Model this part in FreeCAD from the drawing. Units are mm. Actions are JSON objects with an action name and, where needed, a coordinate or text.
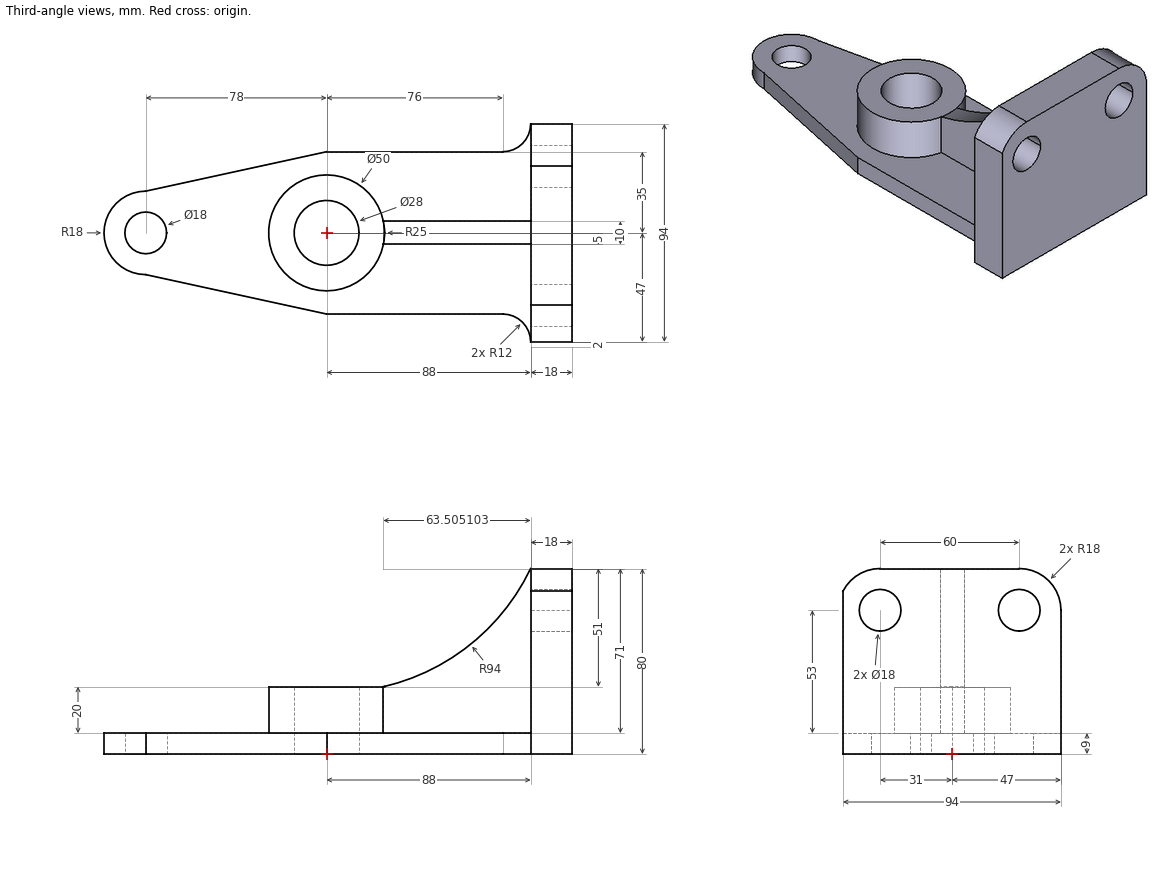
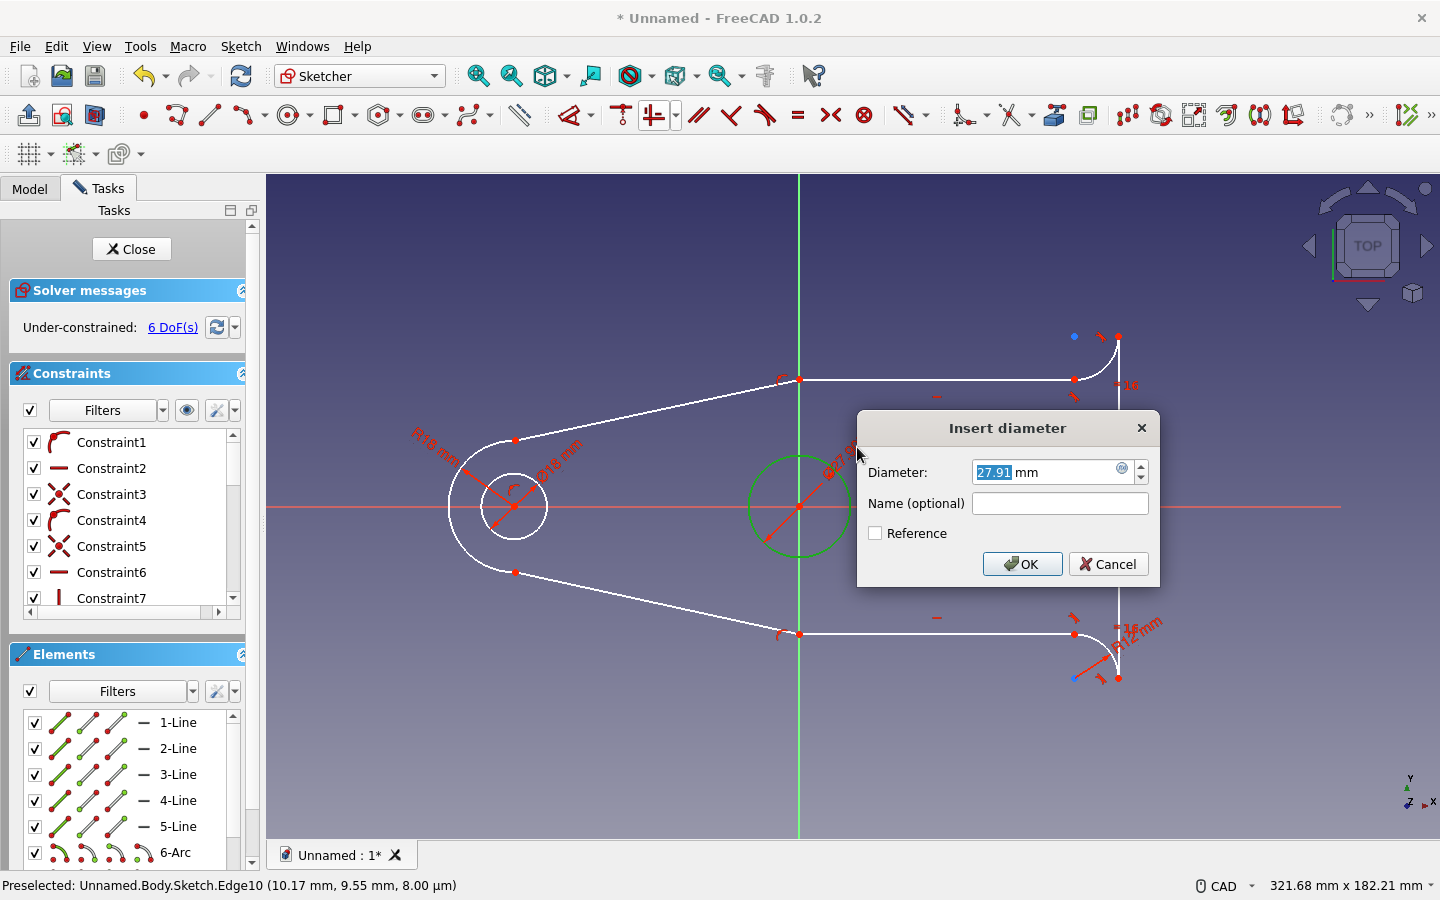
{"action": "type", "text": "28"}
{"action": "key", "text": "Return"}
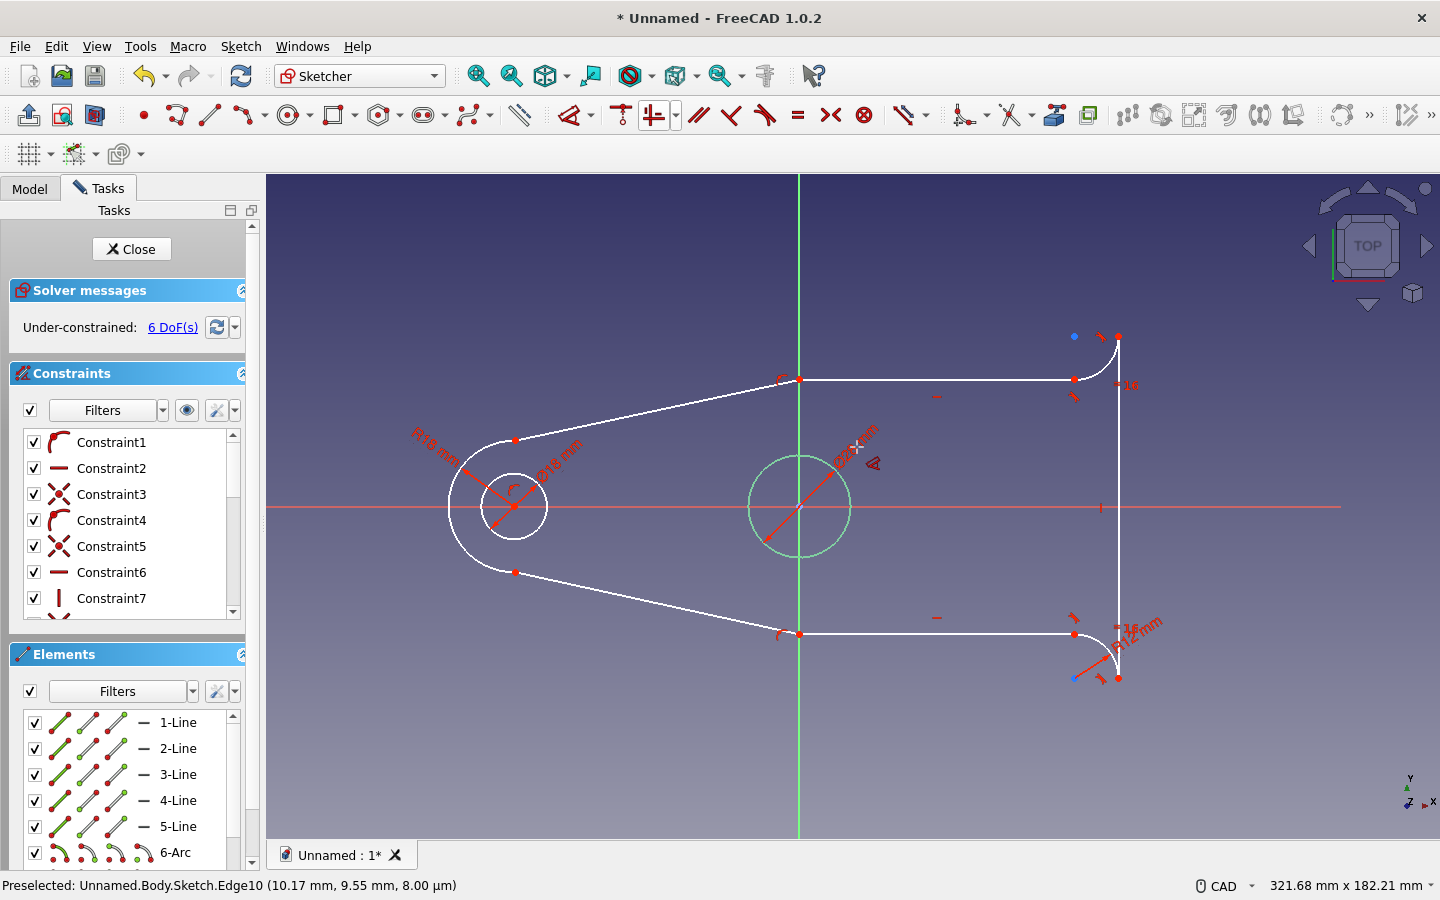
{"action": "left_click", "coordinate": [992, 380]}
{"action": "left_click", "coordinate": [937, 346]}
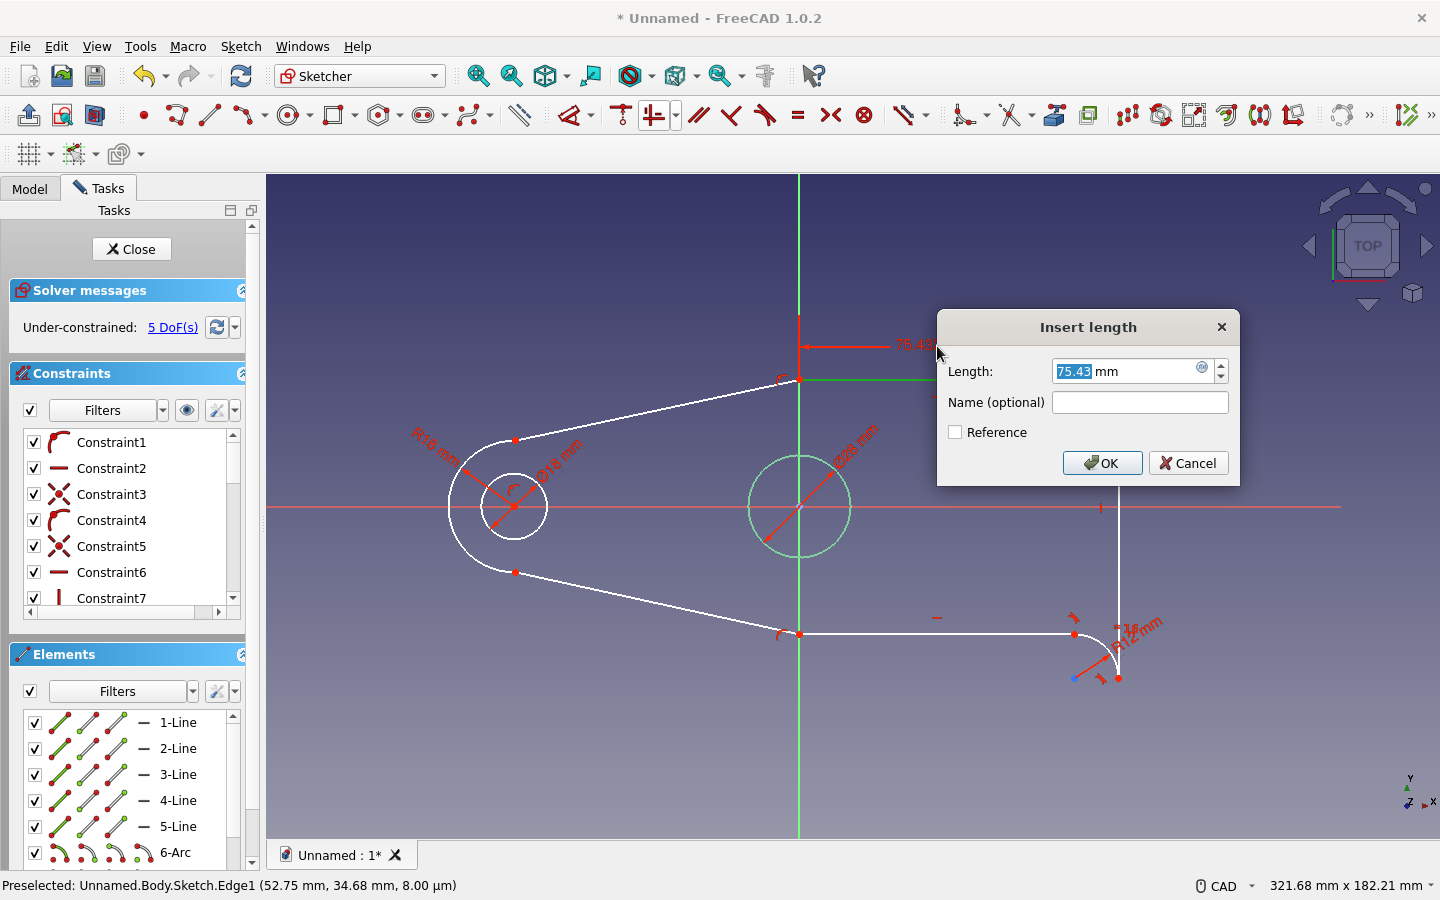
{"action": "type", "text": "76"}
{"action": "key", "text": "Return"}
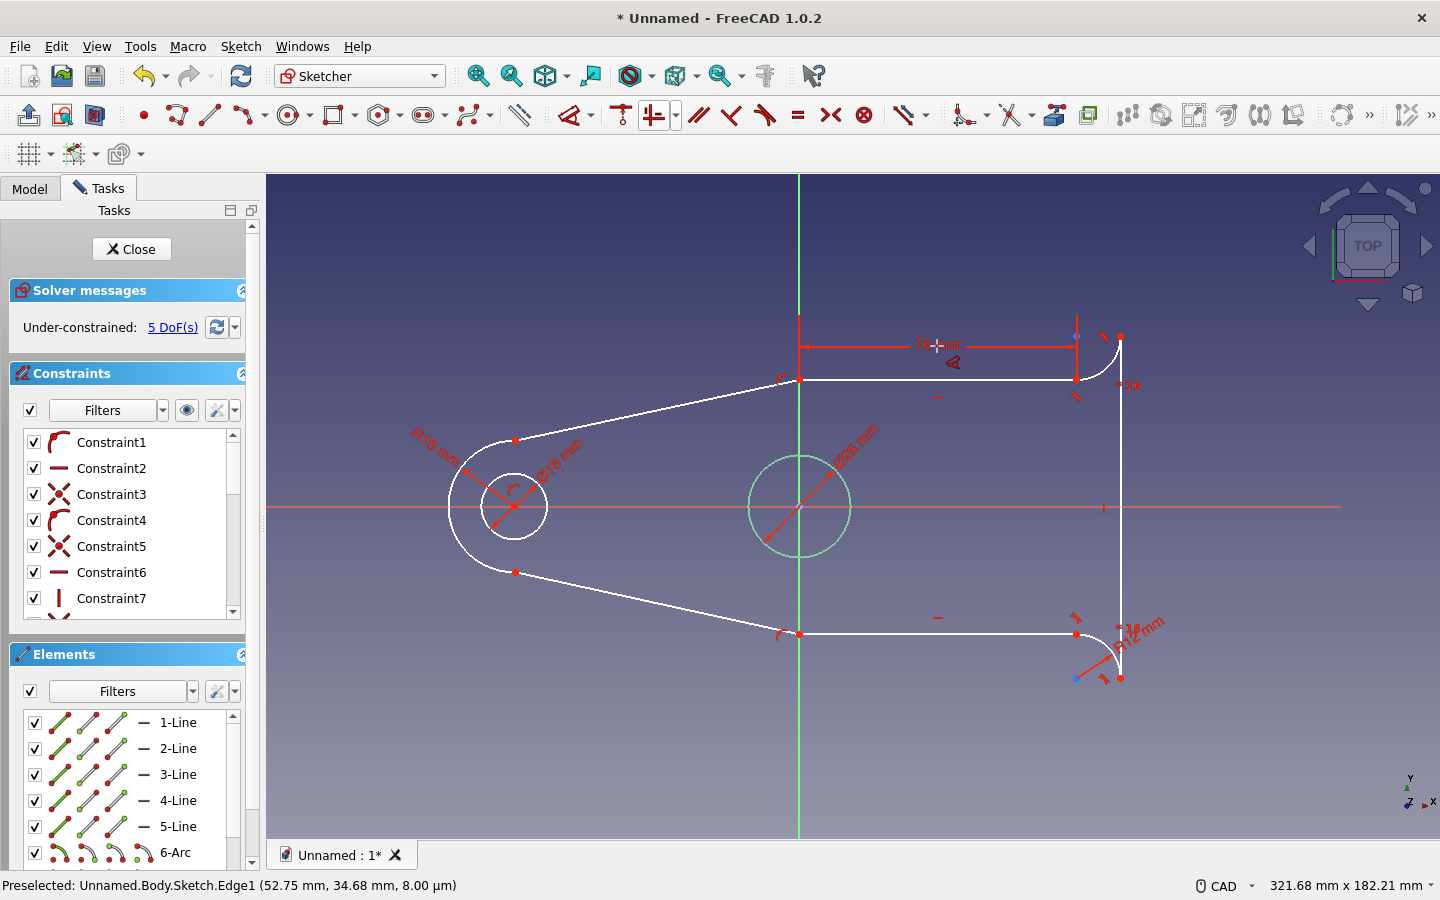
{"action": "left_click", "coordinate": [1121, 576]}
{"action": "left_click", "coordinate": [1155, 429]}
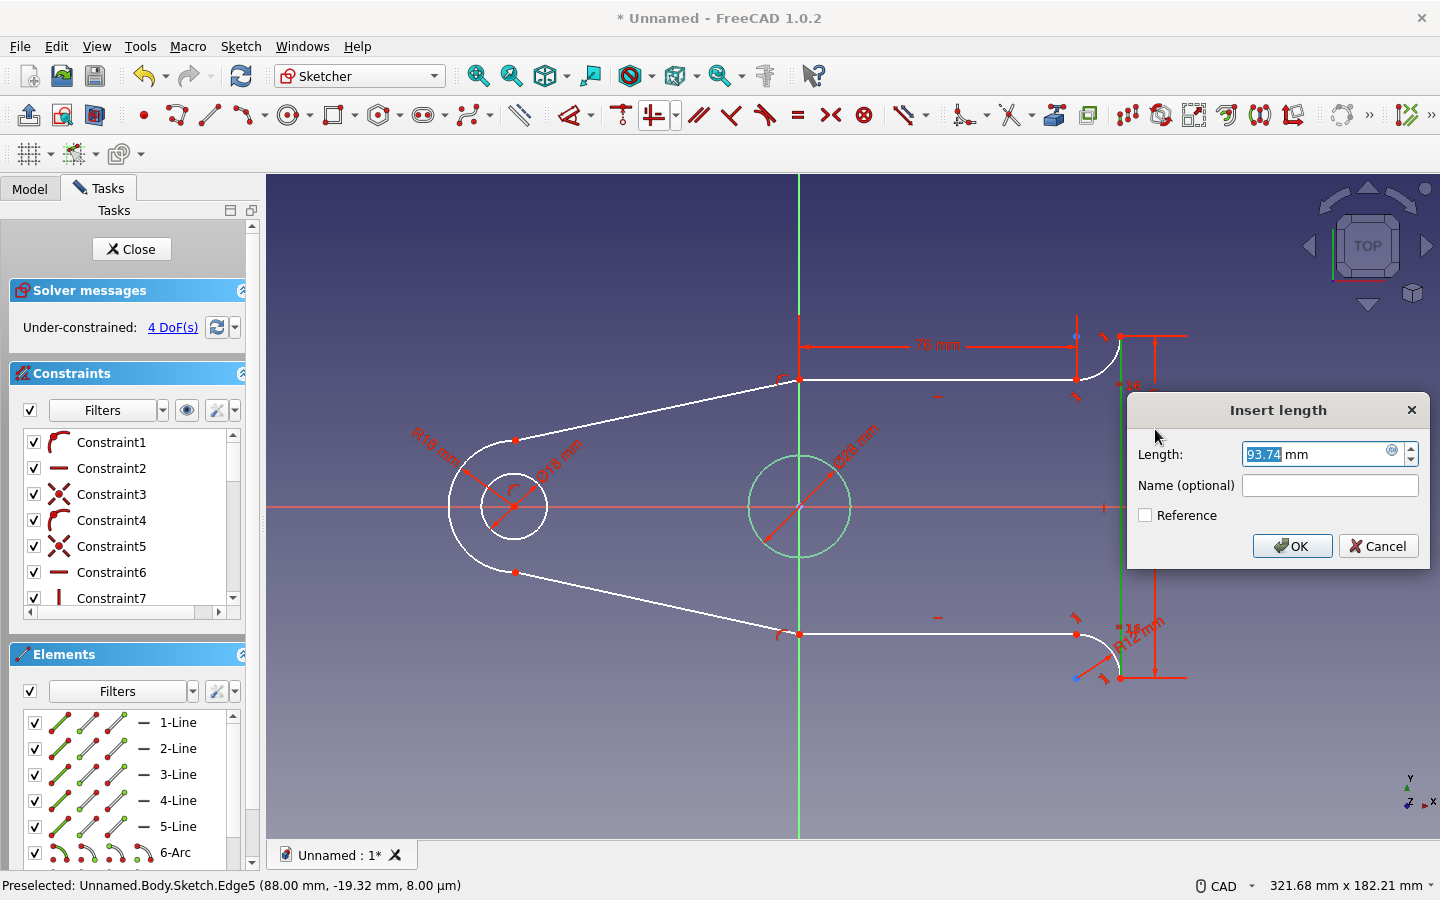
{"action": "type", "text": "94"}
{"action": "key", "text": "Return"}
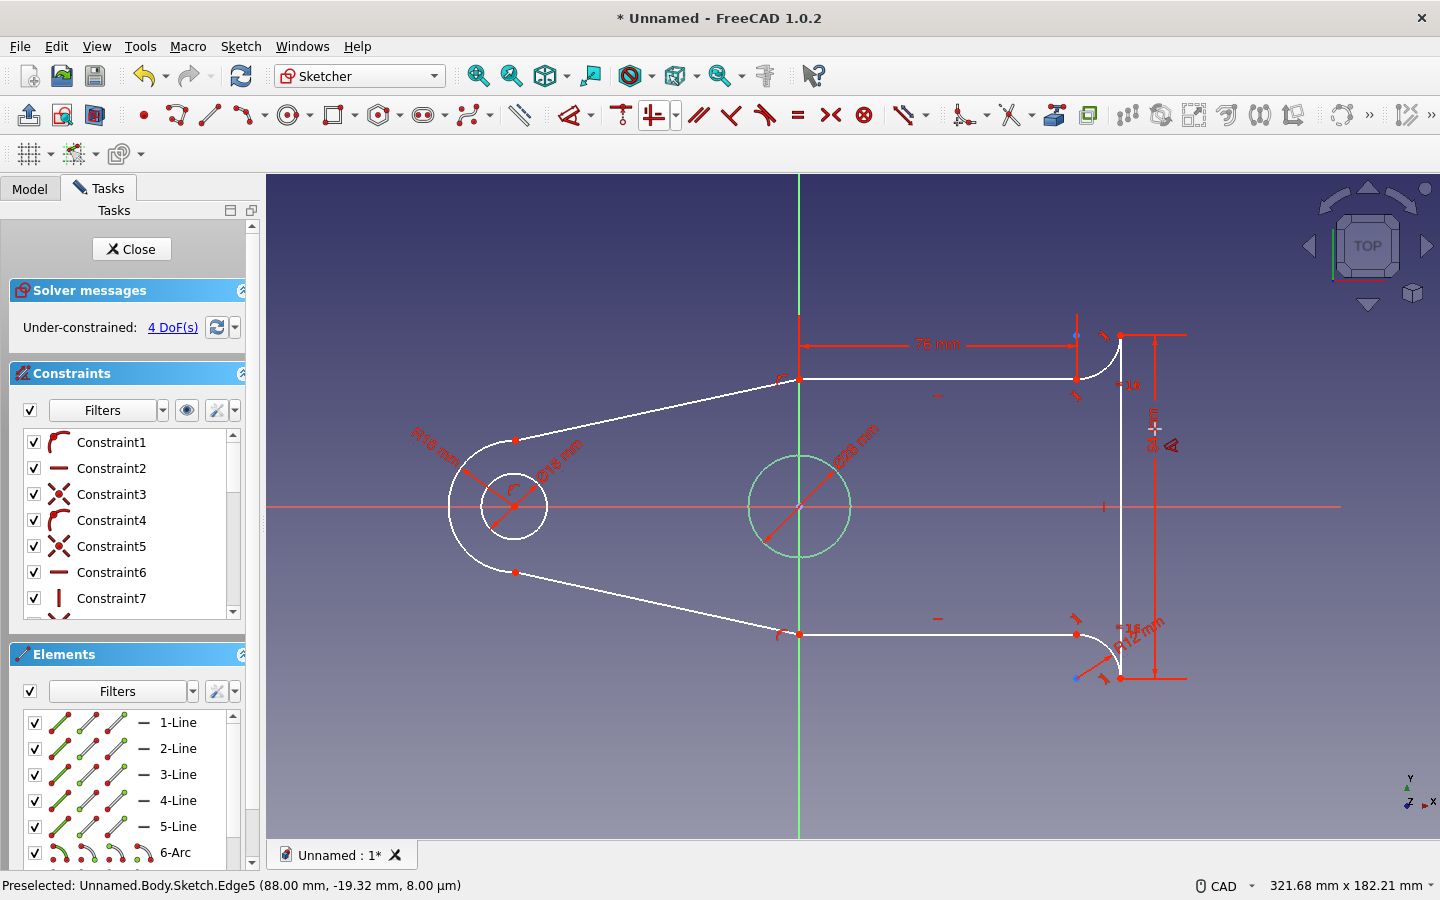
{"action": "left_click", "coordinate": [514, 507]}
{"action": "left_click", "coordinate": [657, 541]}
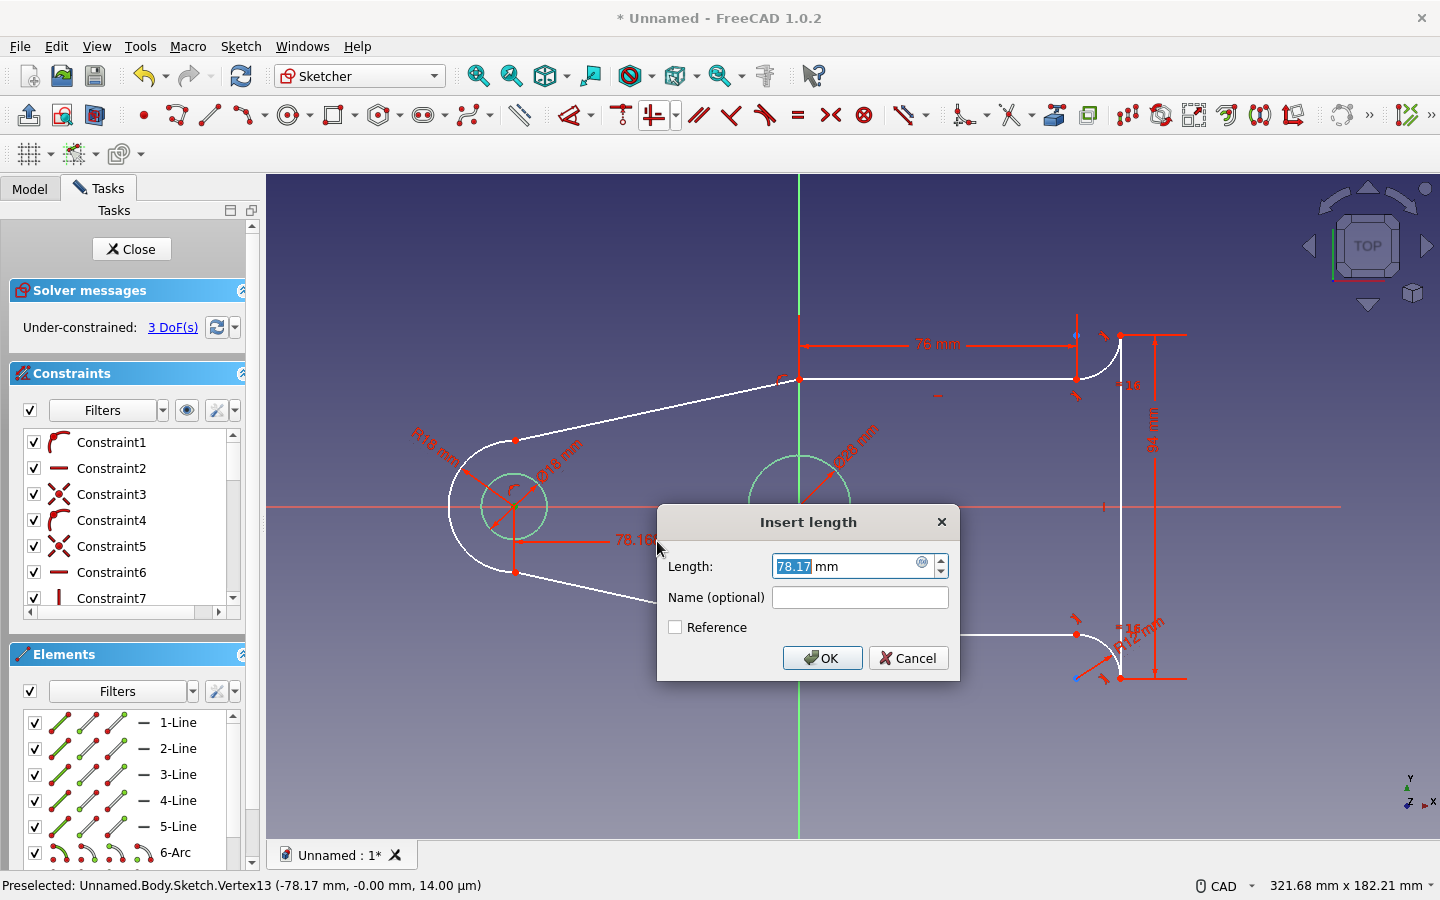
{"action": "type", "text": "78"}
{"action": "key", "text": "Return"}